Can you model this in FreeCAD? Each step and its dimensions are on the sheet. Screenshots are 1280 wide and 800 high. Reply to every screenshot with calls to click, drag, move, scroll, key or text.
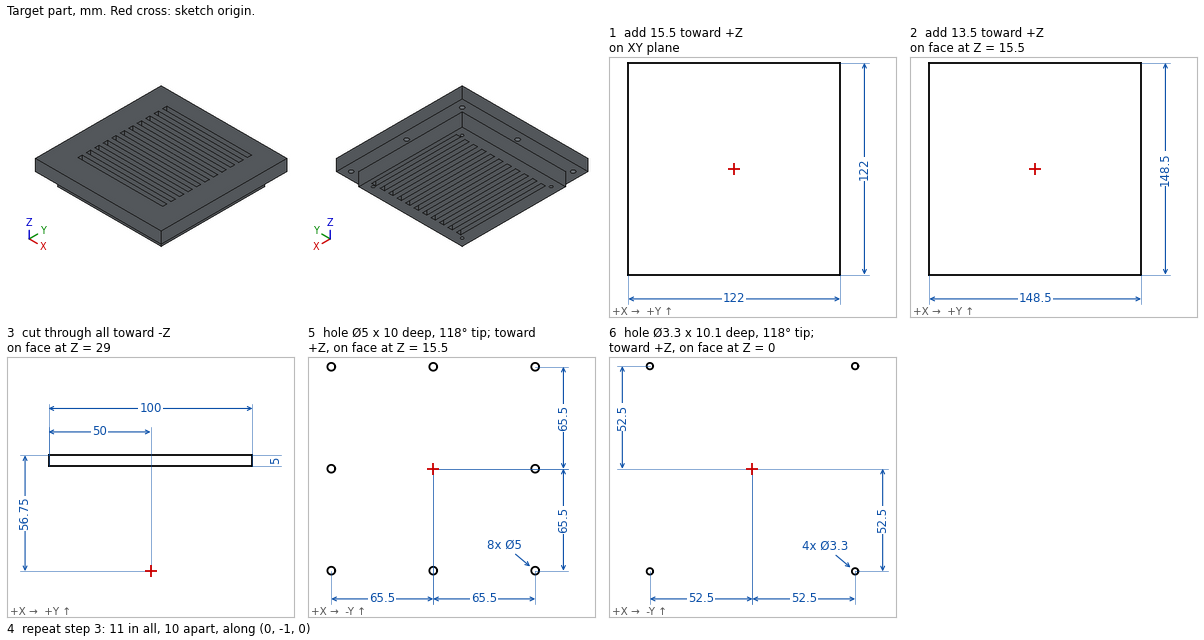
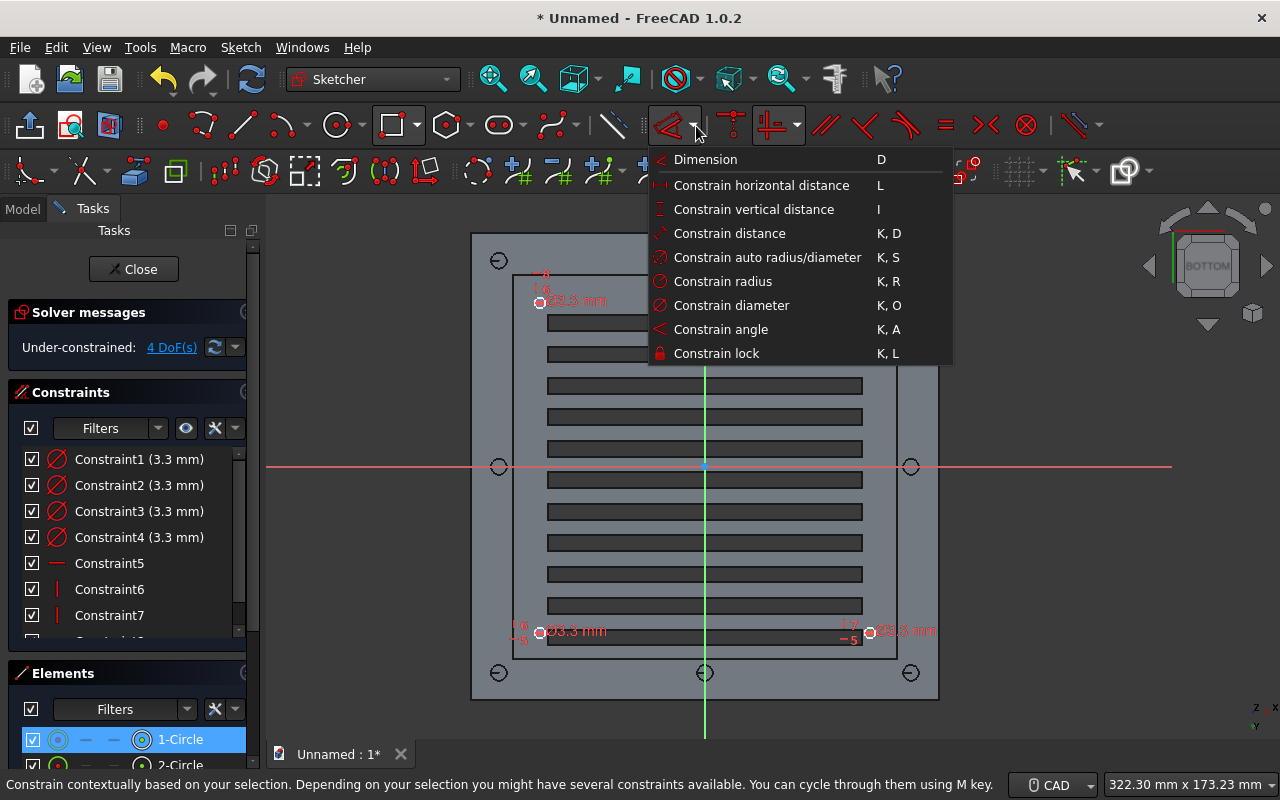
click(801, 185)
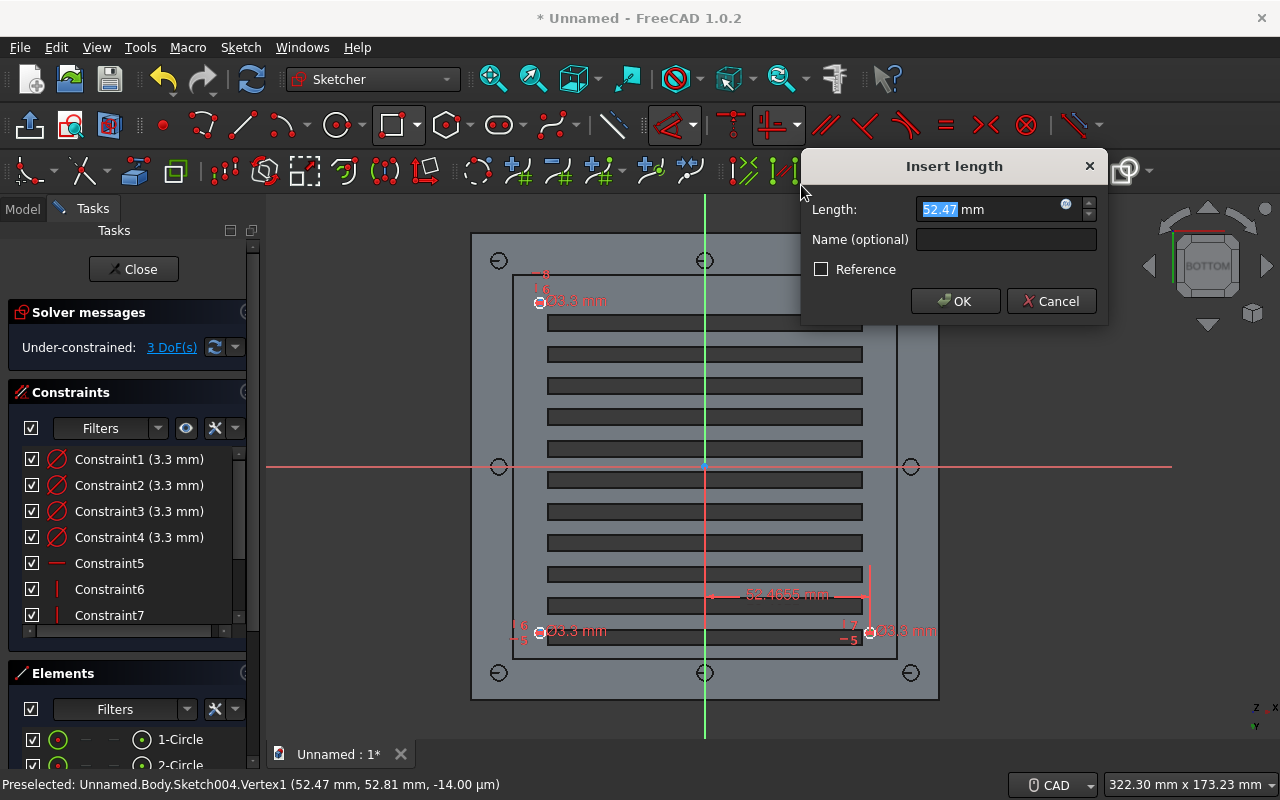
text(52.5)
key(Return)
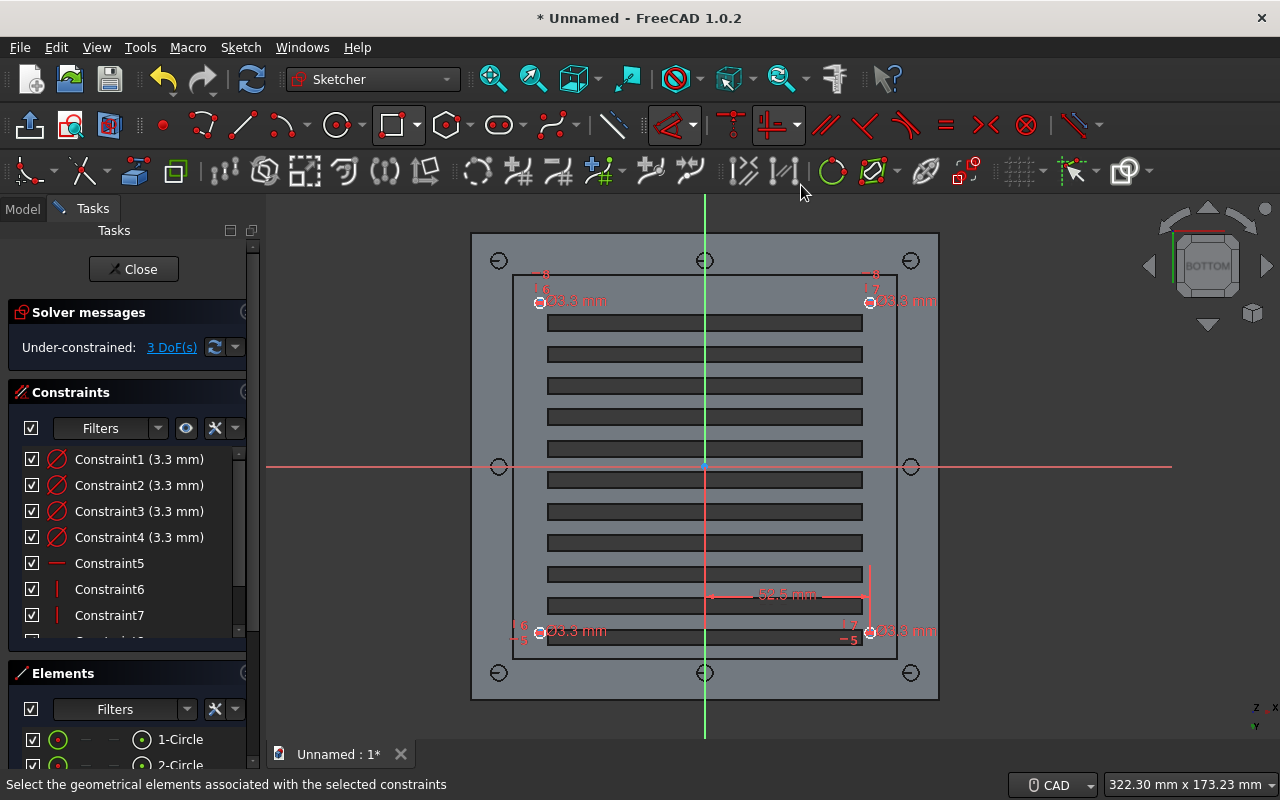
click(870, 633)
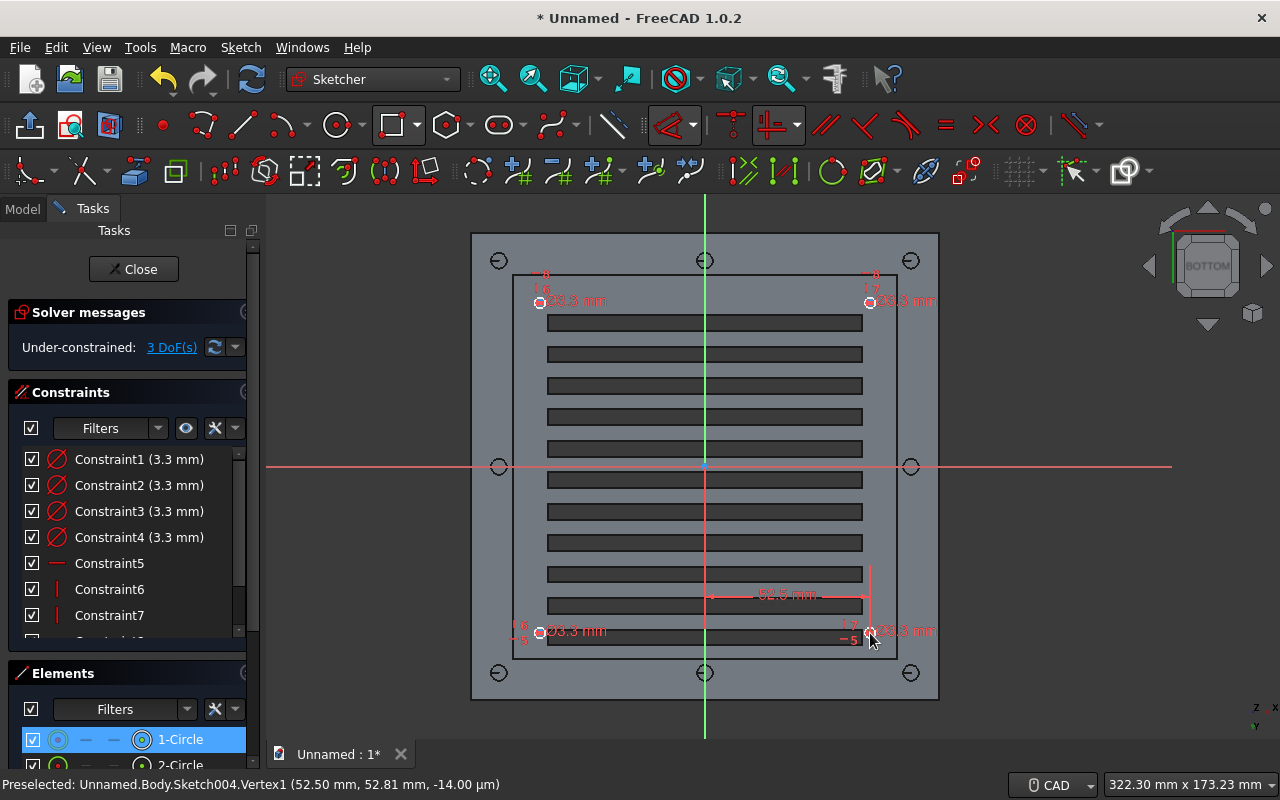
key(i)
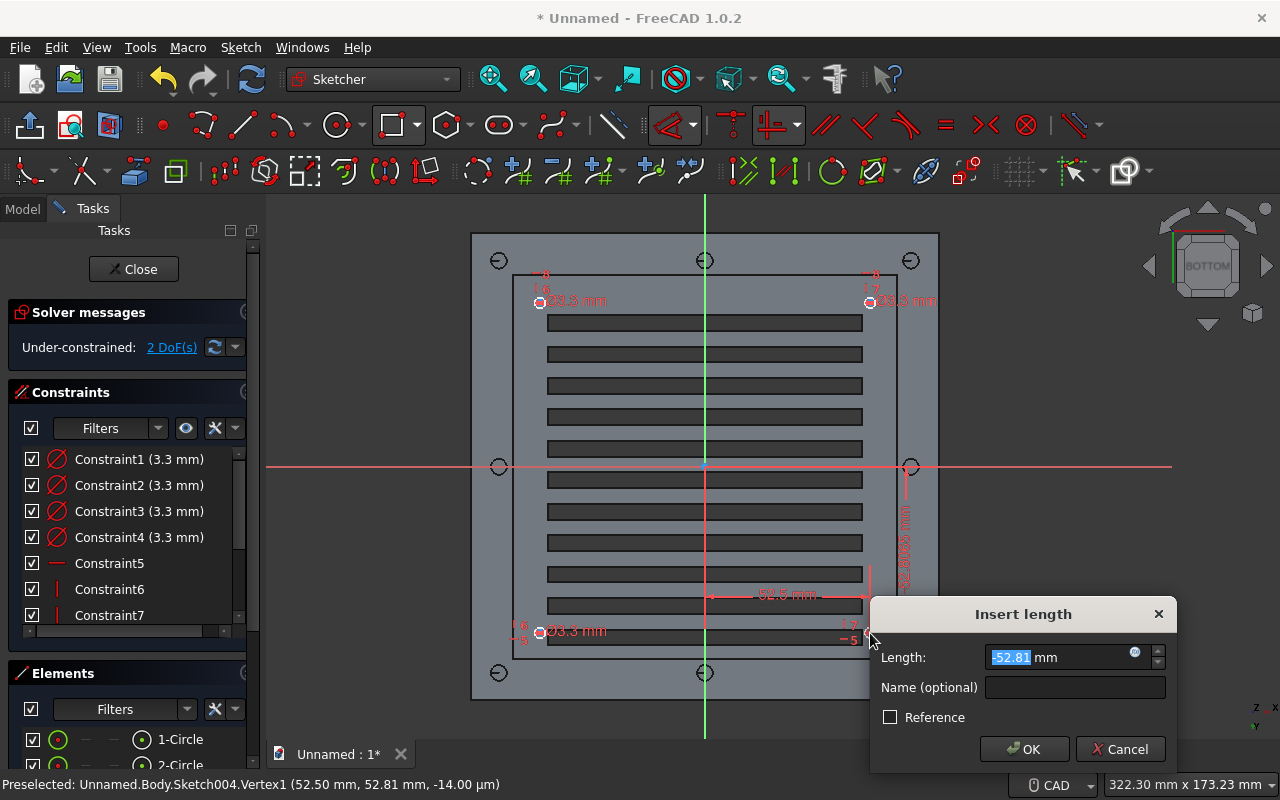
text(-52.5)
key(Return)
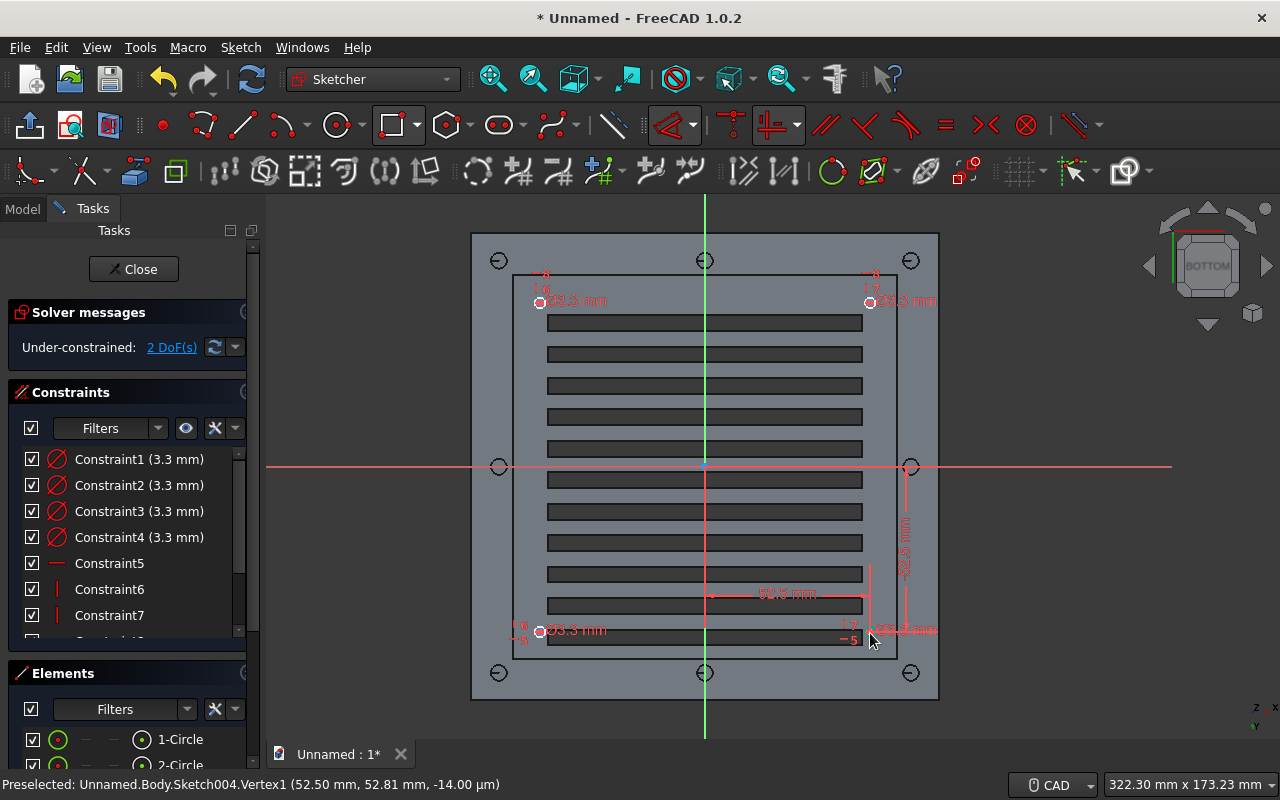
click(540, 632)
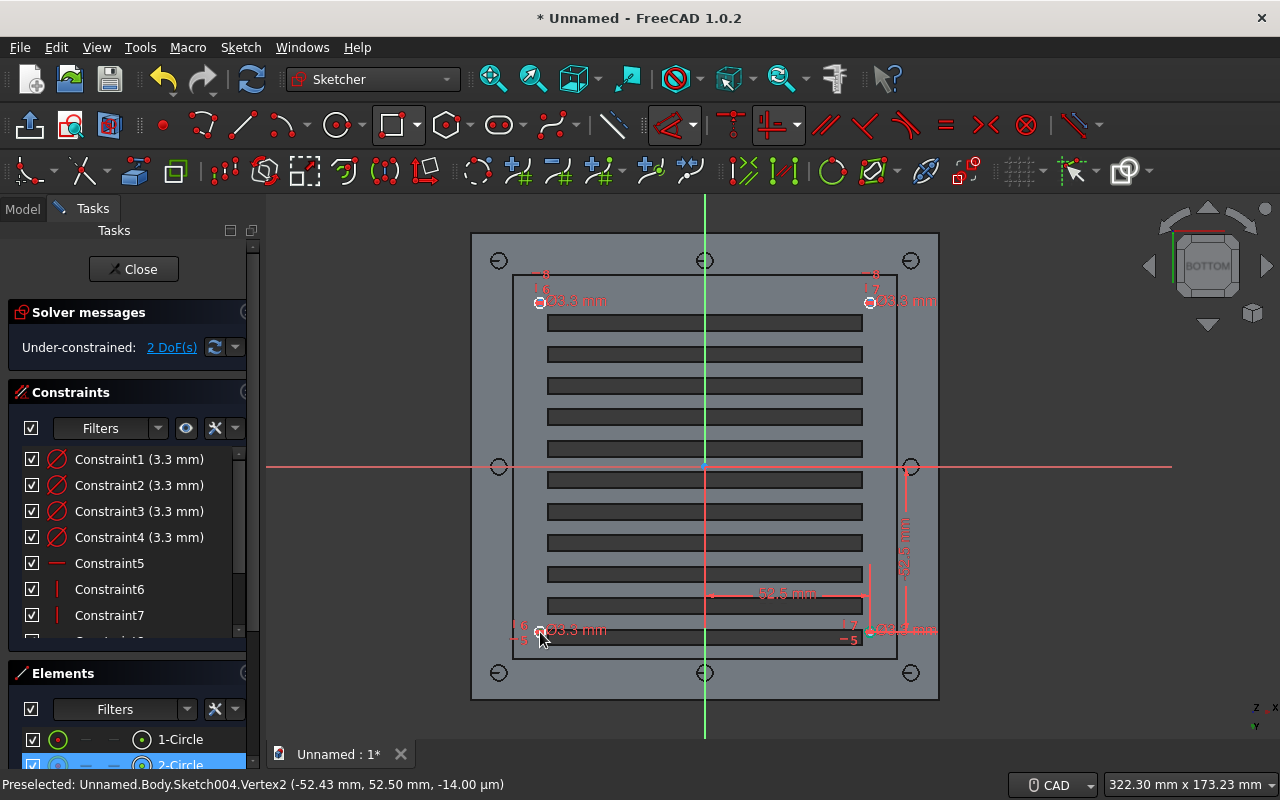
key(l)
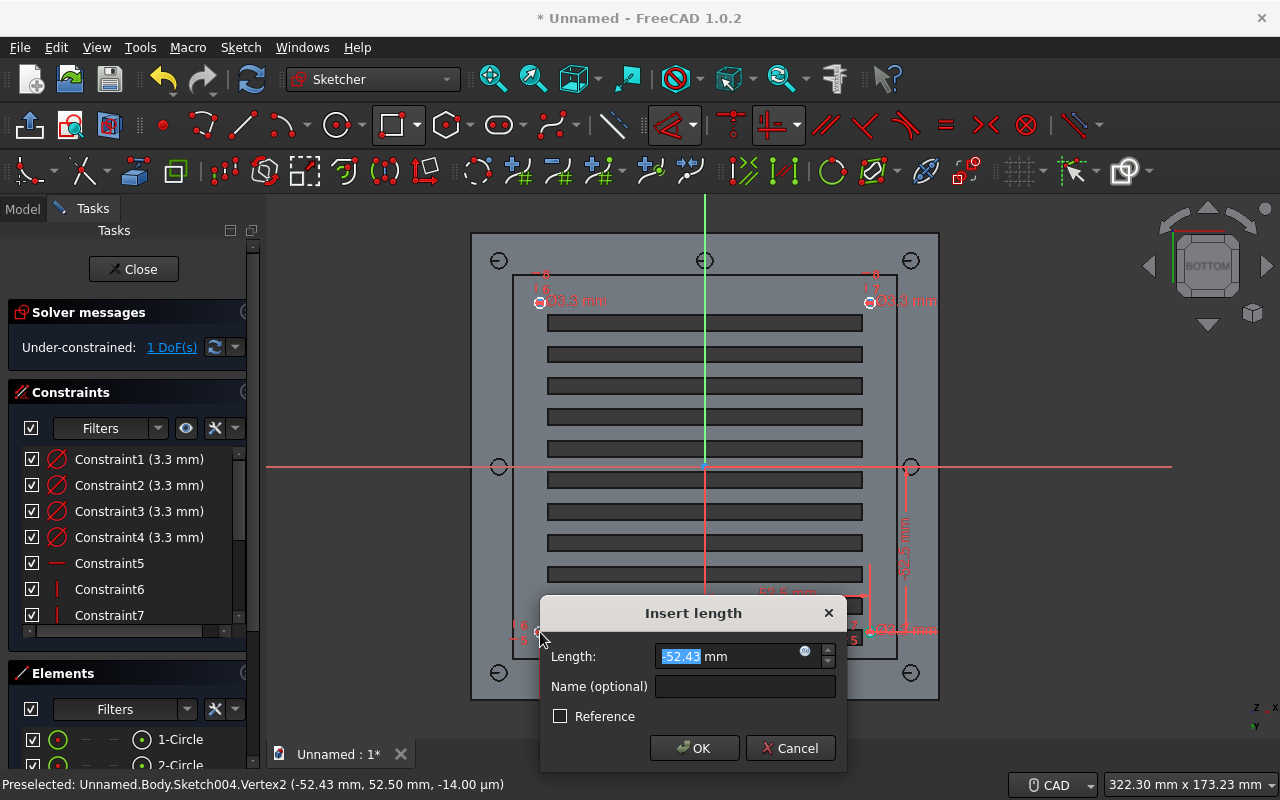
text(-52.5)
key(Return)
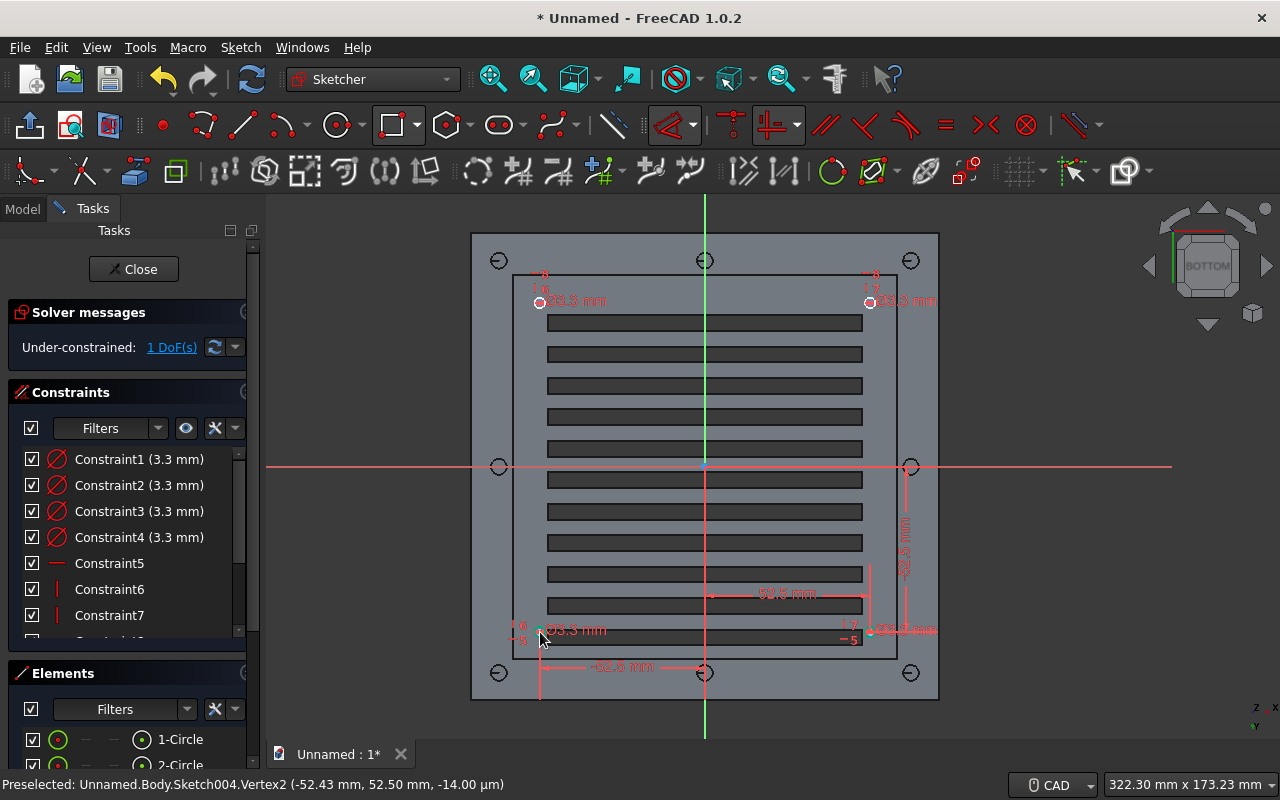
click(540, 303)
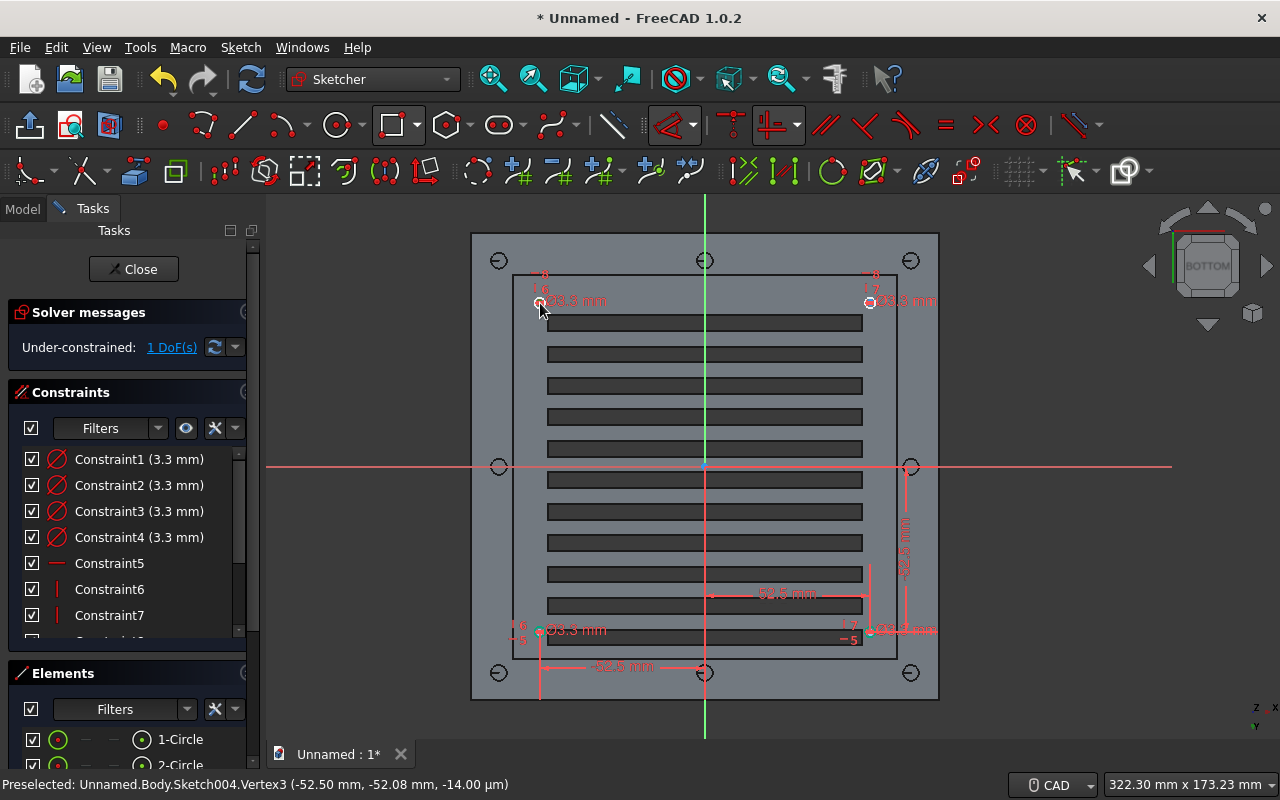
click(696, 126)